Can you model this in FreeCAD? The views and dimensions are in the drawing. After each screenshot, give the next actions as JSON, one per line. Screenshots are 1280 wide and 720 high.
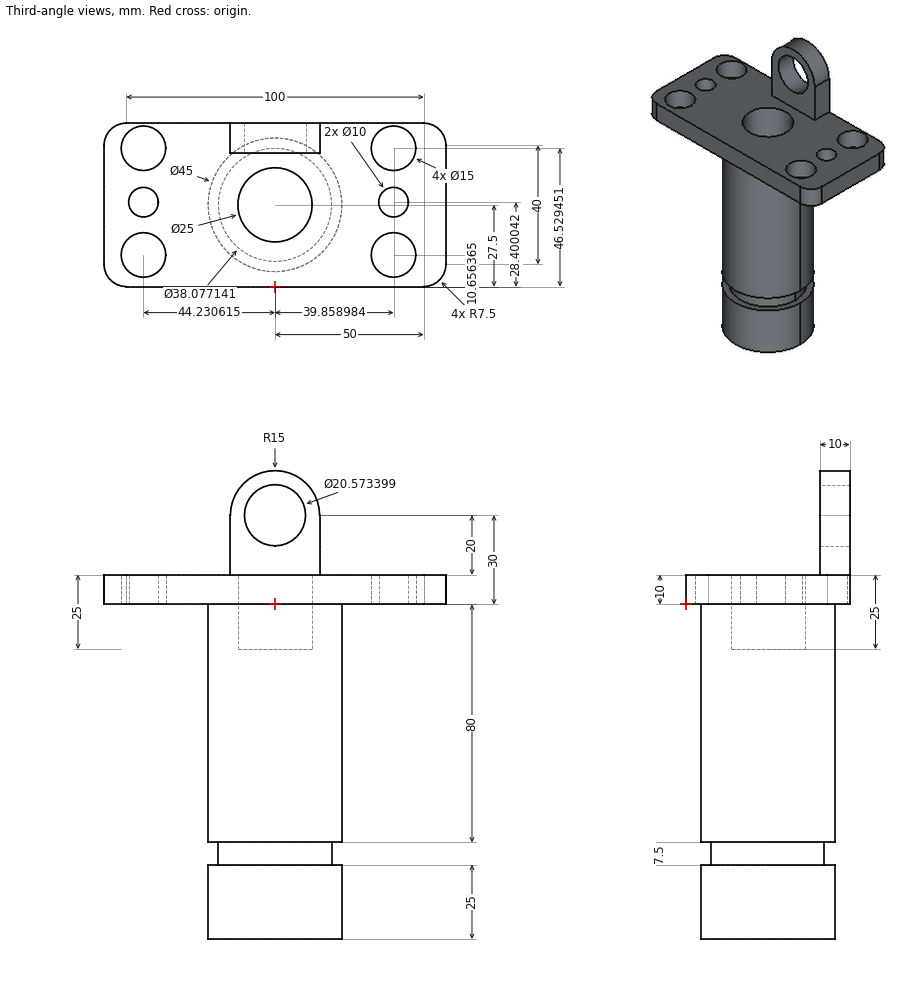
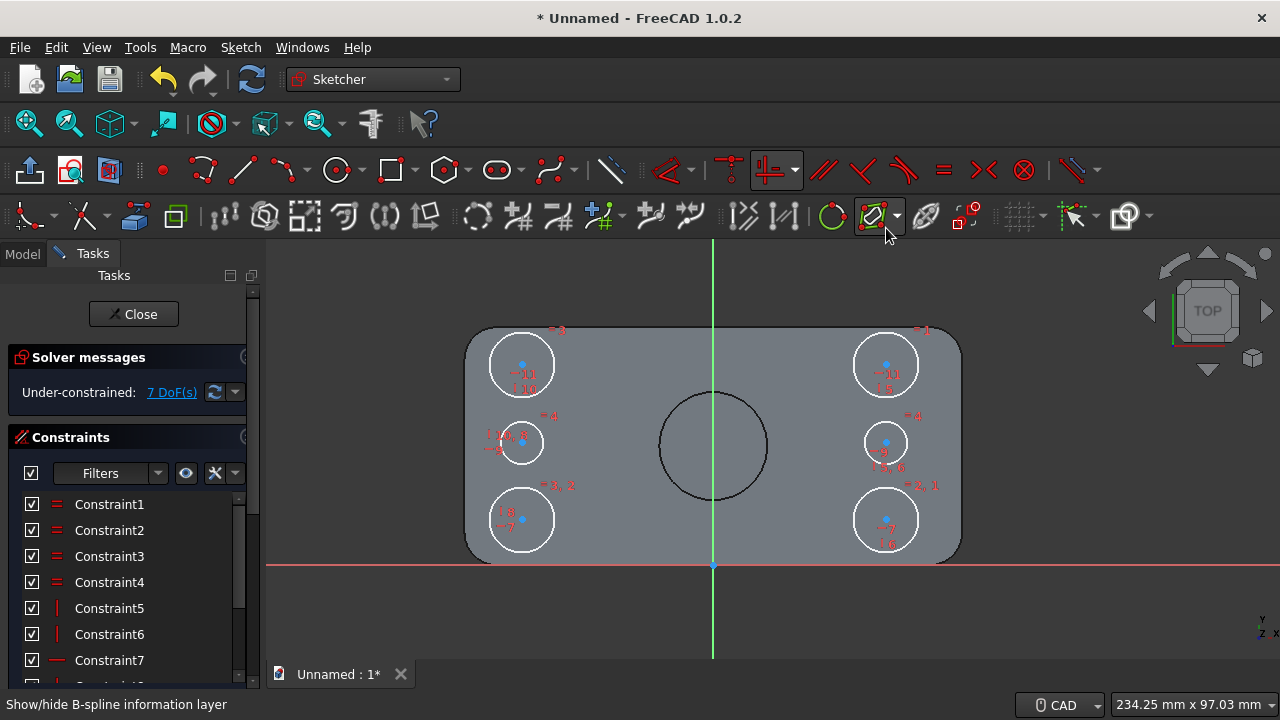
{"action": "left_click", "coordinate": [666, 170]}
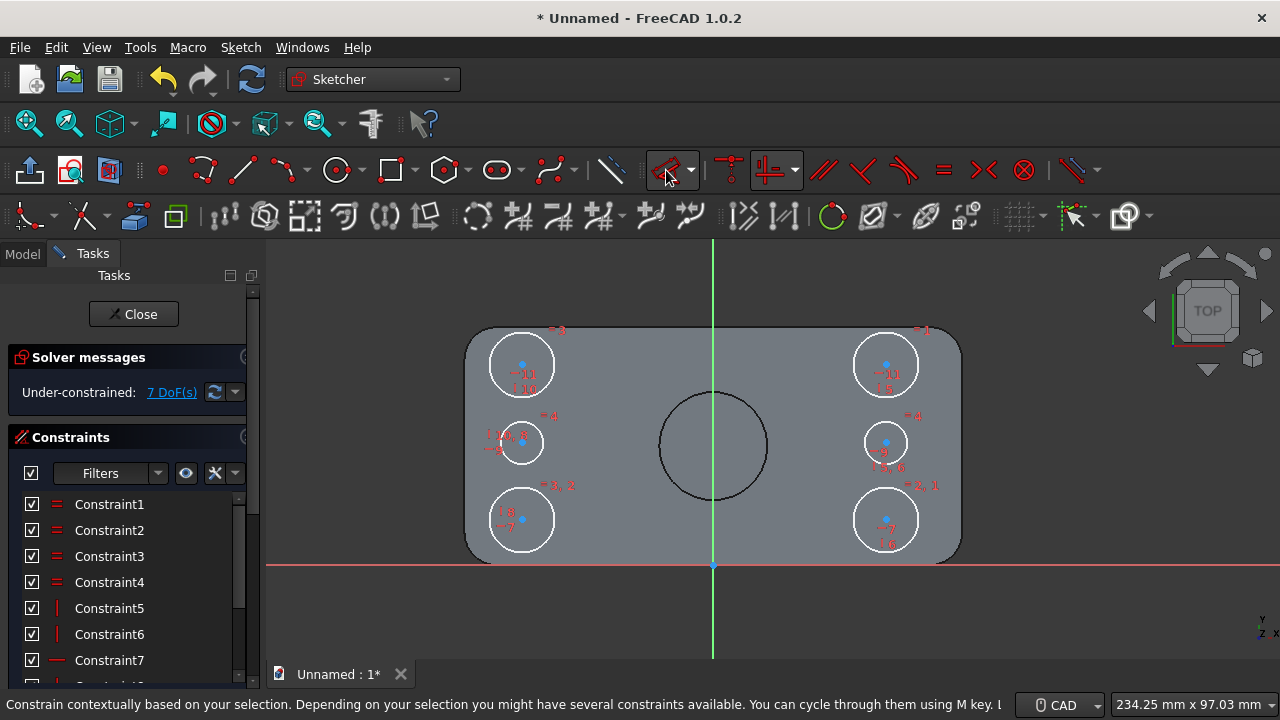
{"action": "left_click", "coordinate": [909, 342]}
{"action": "left_click", "coordinate": [932, 319]}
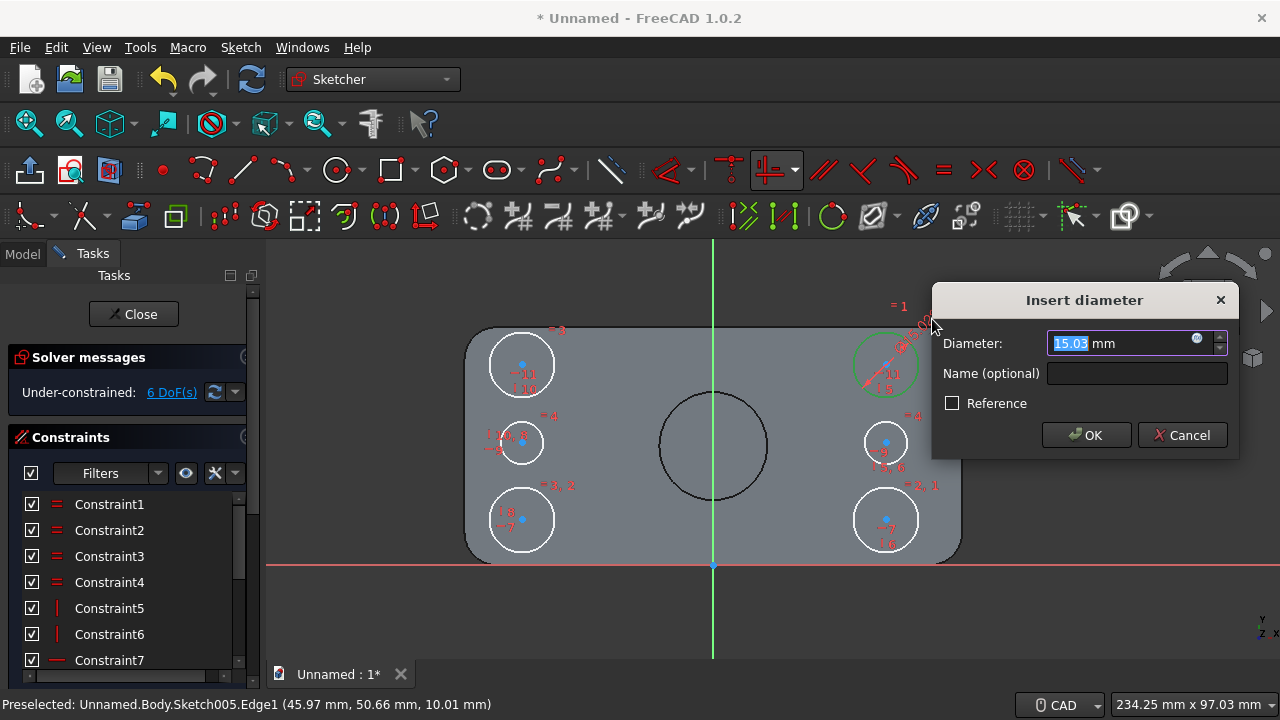
{"action": "type", "text": "15"}
{"action": "key", "text": "Return"}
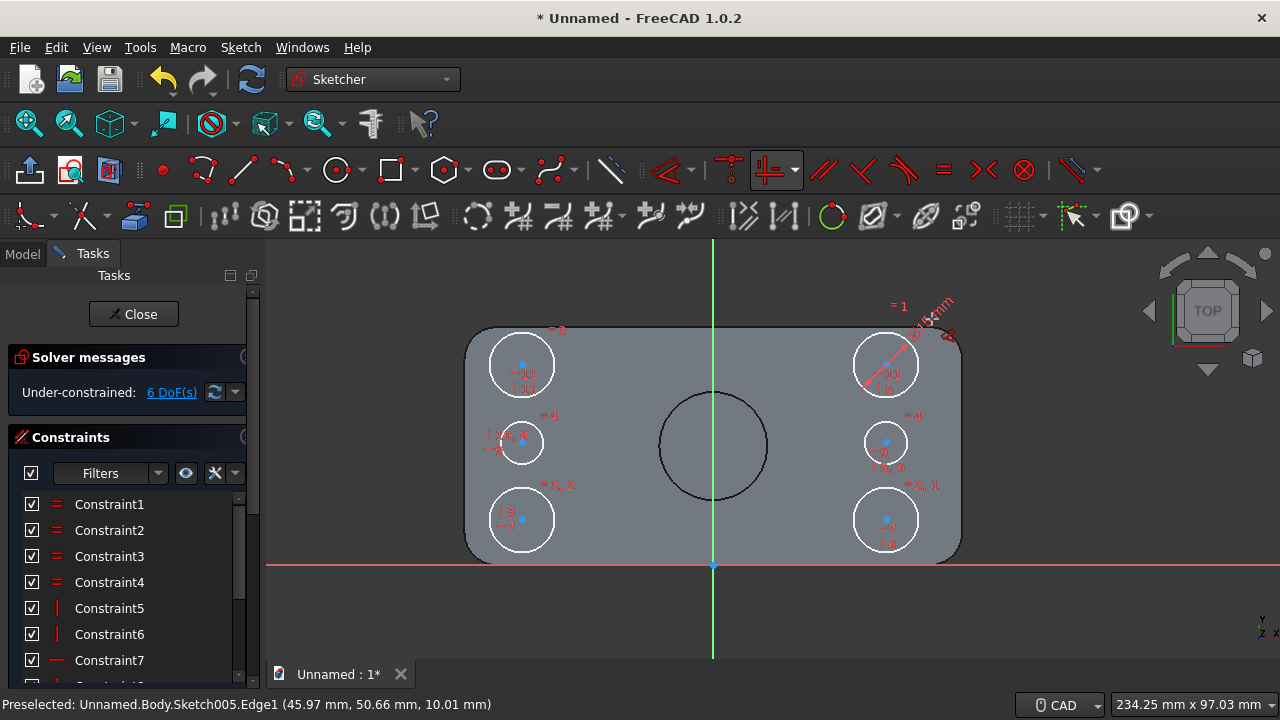
{"action": "left_click", "coordinate": [901, 428]}
{"action": "left_click", "coordinate": [924, 405]}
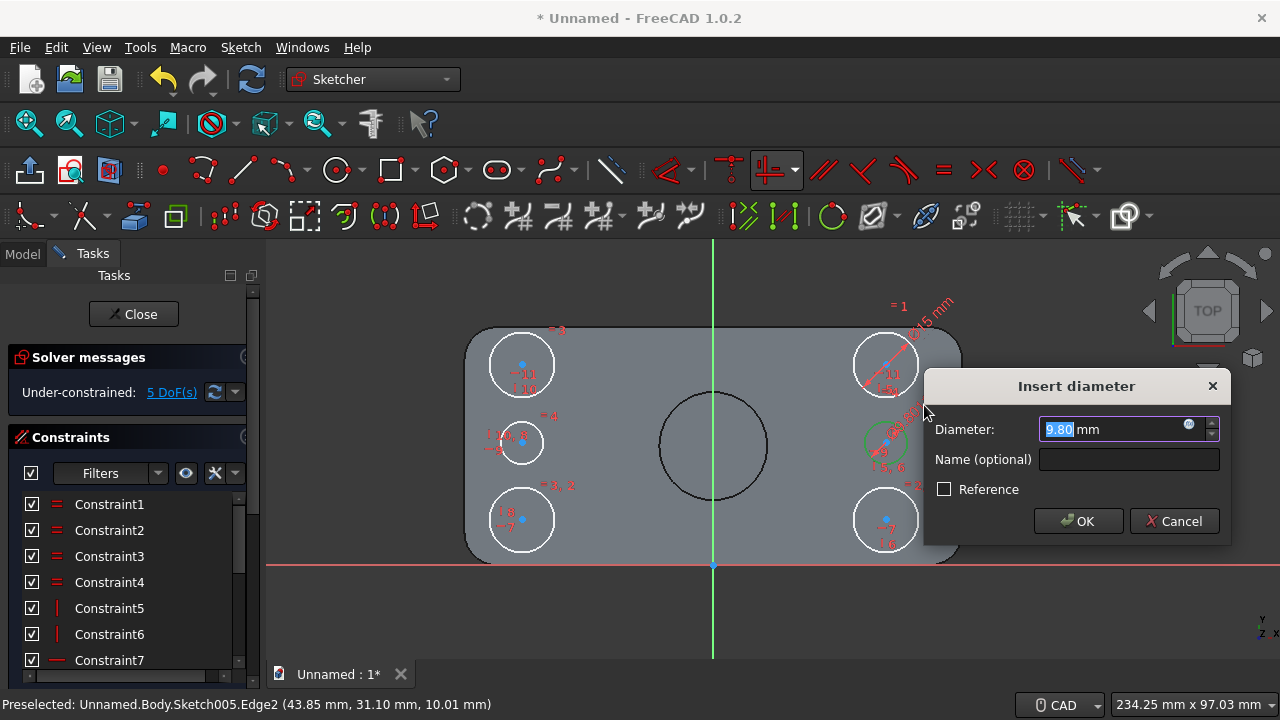
{"action": "type", "text": "10"}
{"action": "key", "text": "Return"}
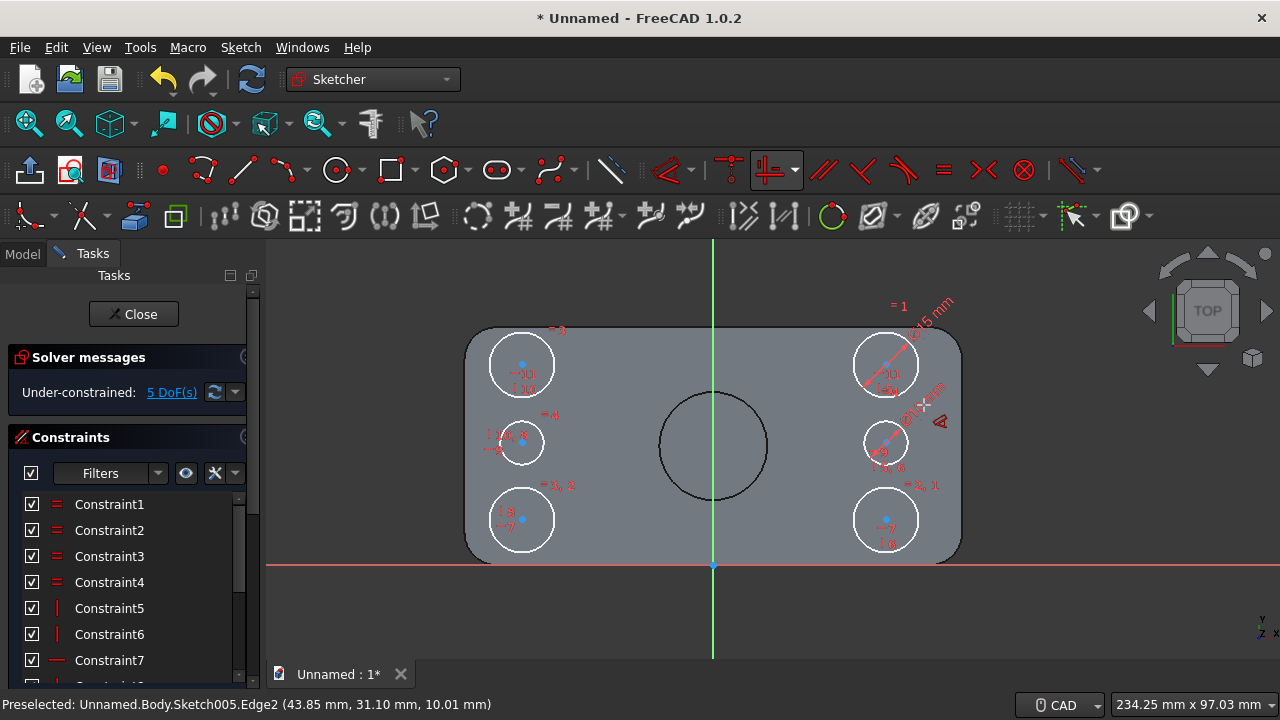
{"action": "left_click", "coordinate": [886, 365]}
{"action": "left_click", "coordinate": [800, 599]}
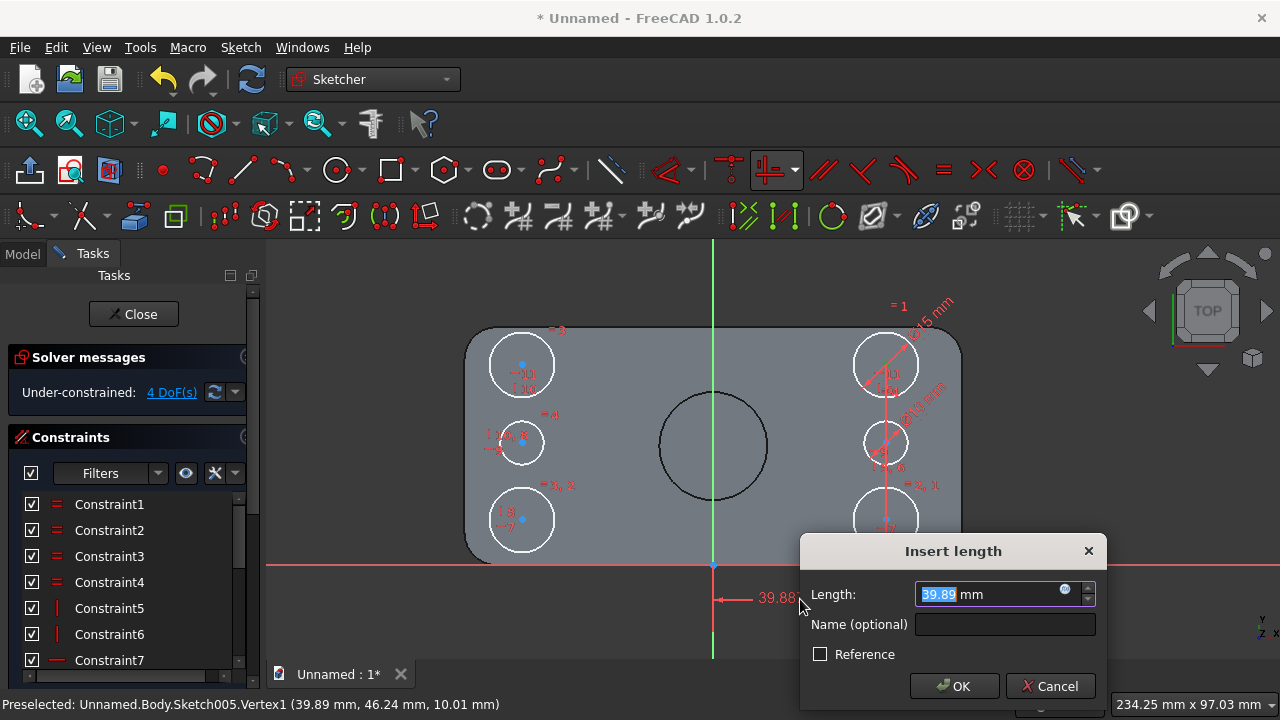
{"action": "type", "text": "39.858984"}
{"action": "key", "text": "Return"}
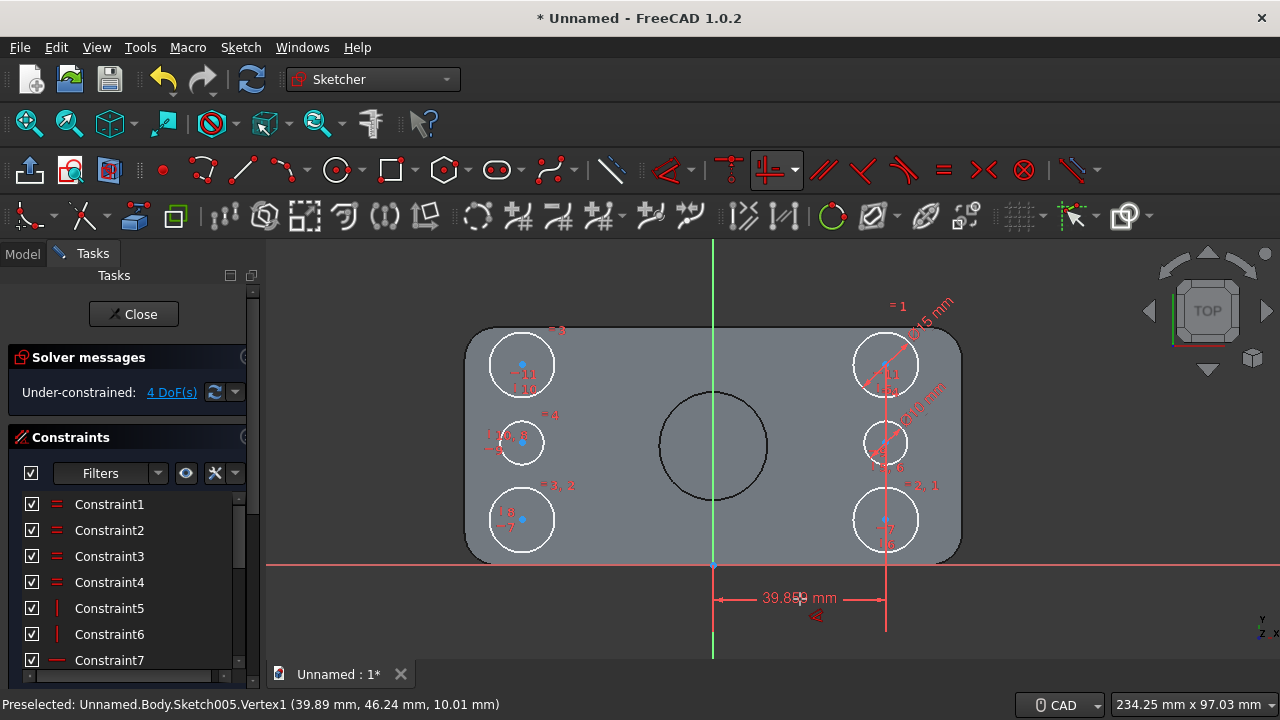
{"action": "left_click", "coordinate": [886, 365]}
{"action": "left_click", "coordinate": [920, 465]}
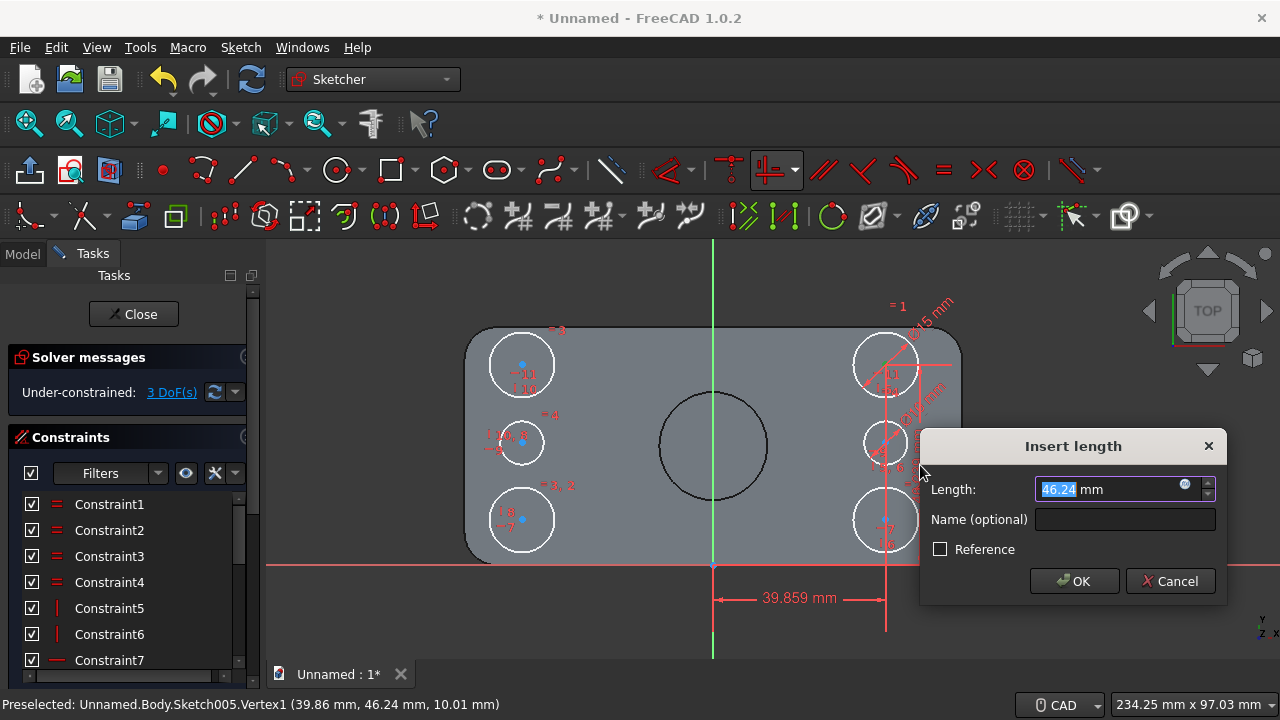
{"action": "type", "text": "46.529451"}
{"action": "key", "text": "Return"}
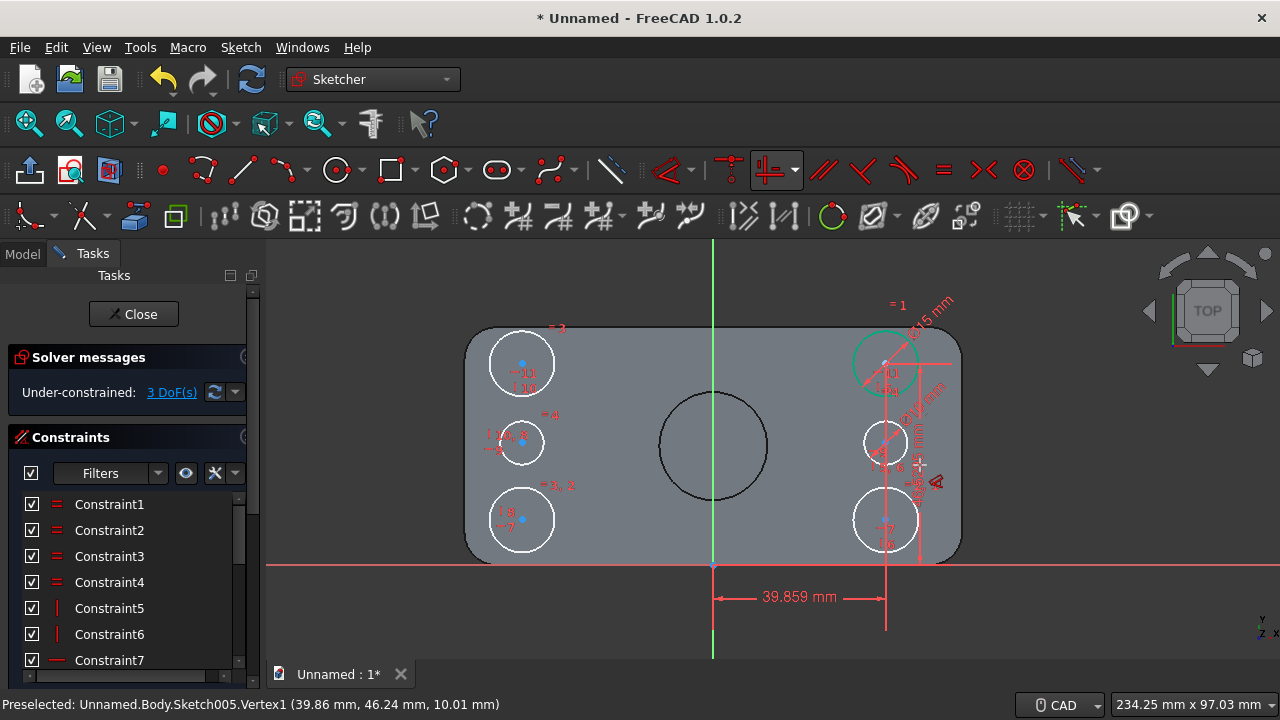
{"action": "left_click", "coordinate": [886, 443]}
{"action": "left_click", "coordinate": [679, 504]}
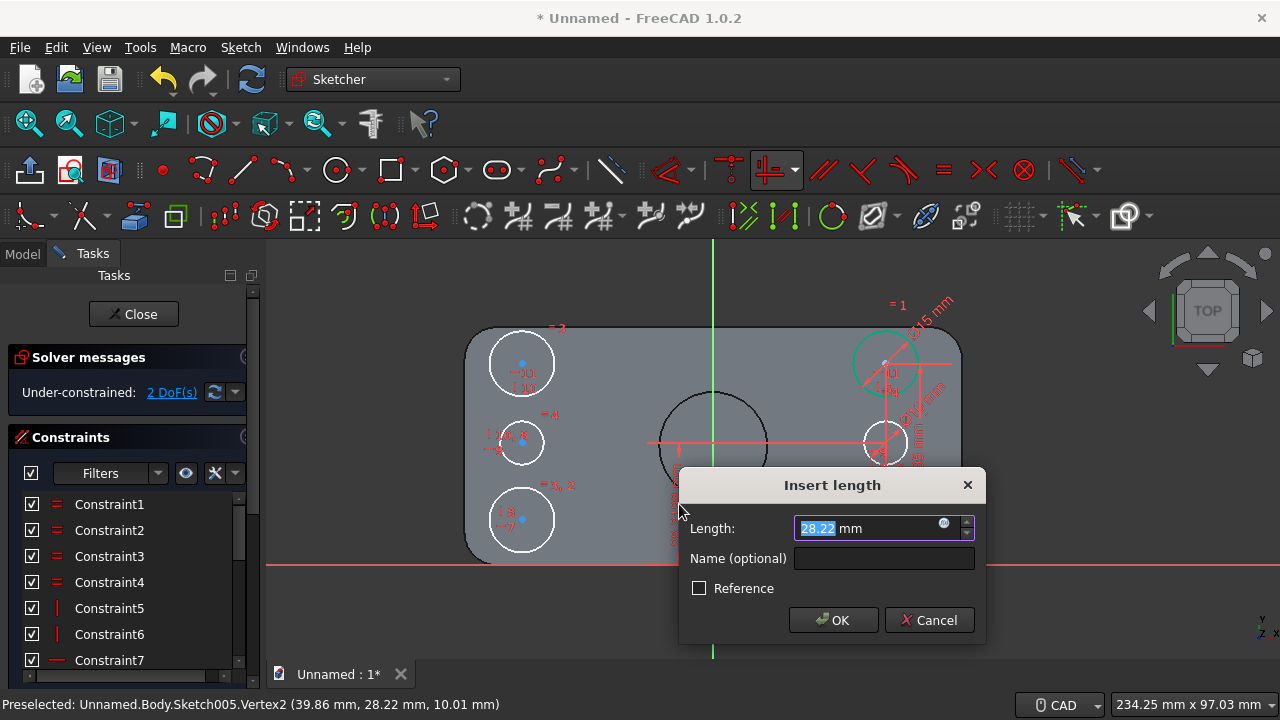
{"action": "type", "text": "28.400042"}
{"action": "key", "text": "Return"}